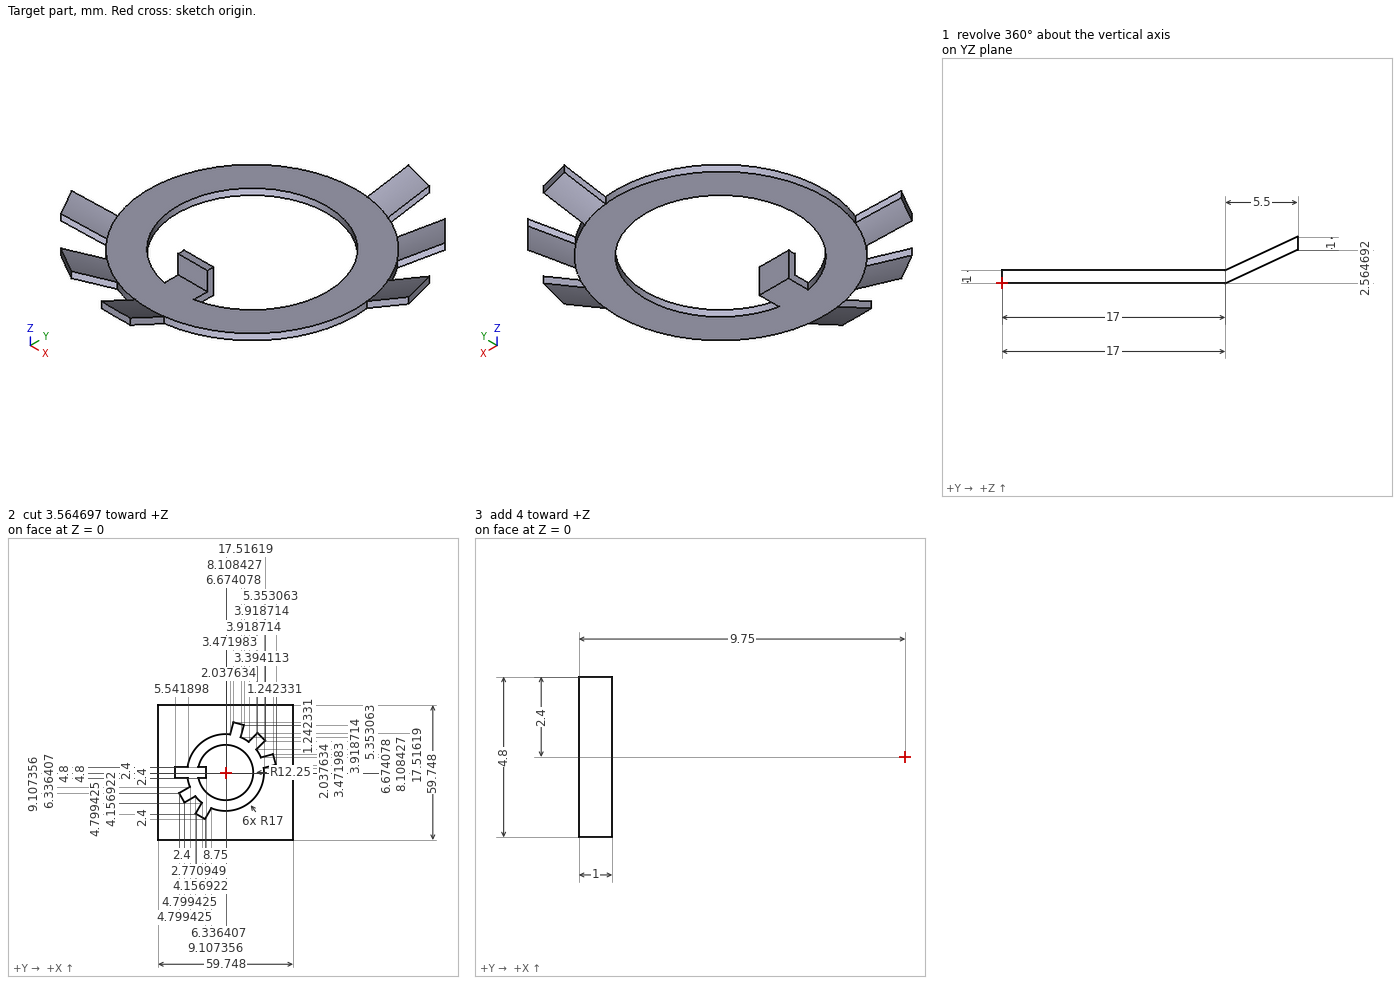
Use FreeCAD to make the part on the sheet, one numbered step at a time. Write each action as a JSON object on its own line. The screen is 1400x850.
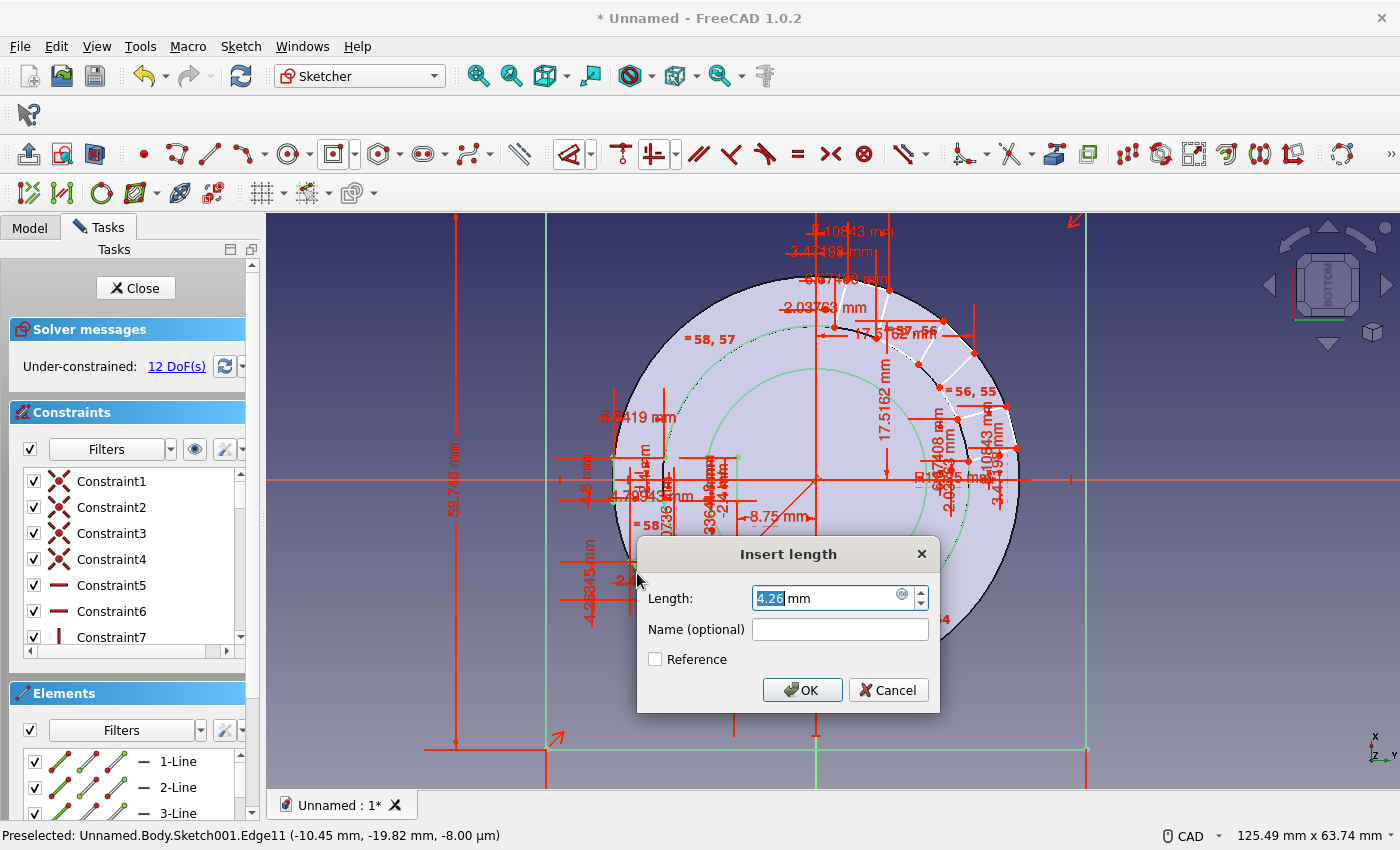
{"action": "type", "text": "4.156922"}
{"action": "key", "text": "Return"}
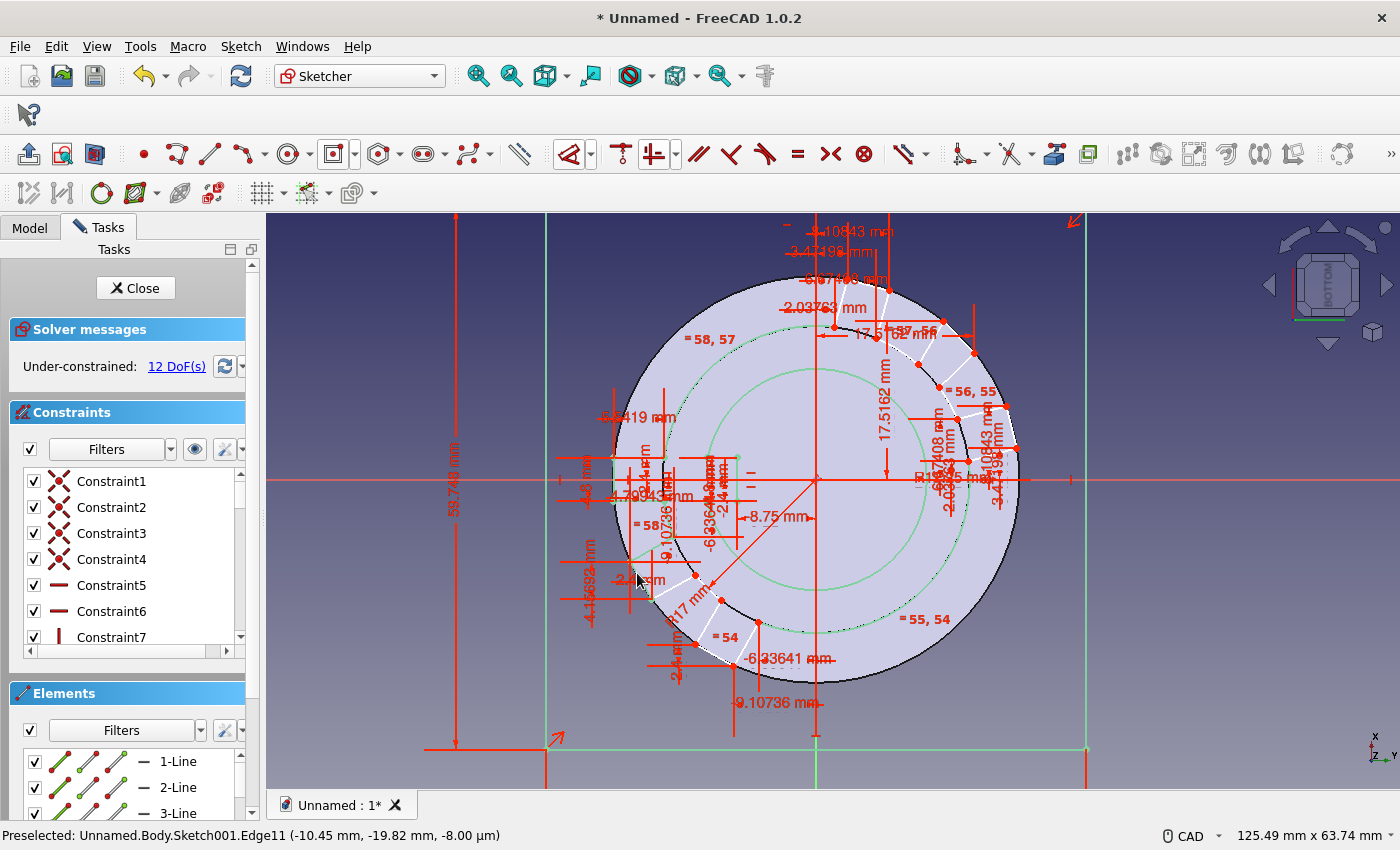
{"action": "left_click", "coordinate": [665, 592]}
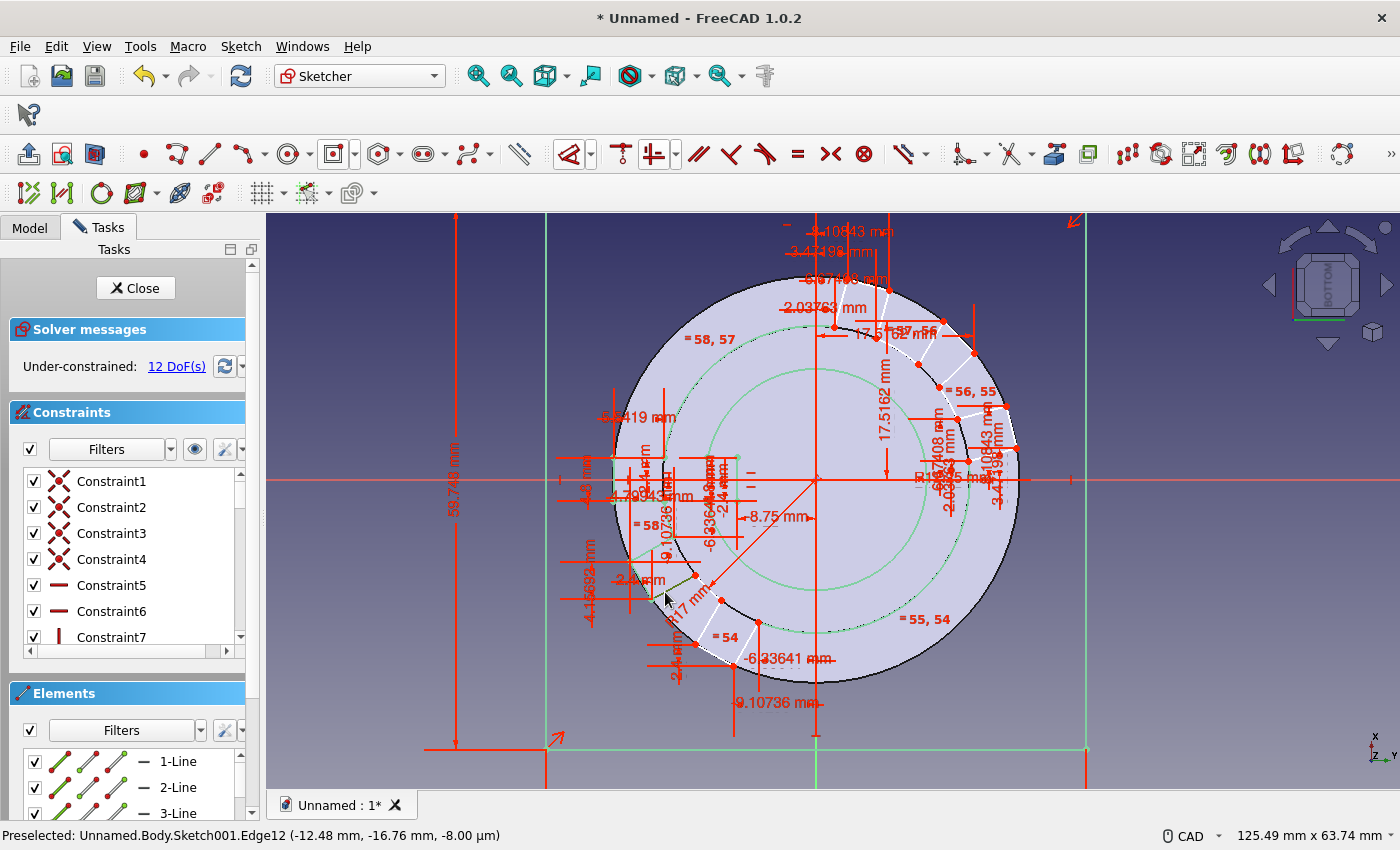
{"action": "left_click", "coordinate": [590, 154]}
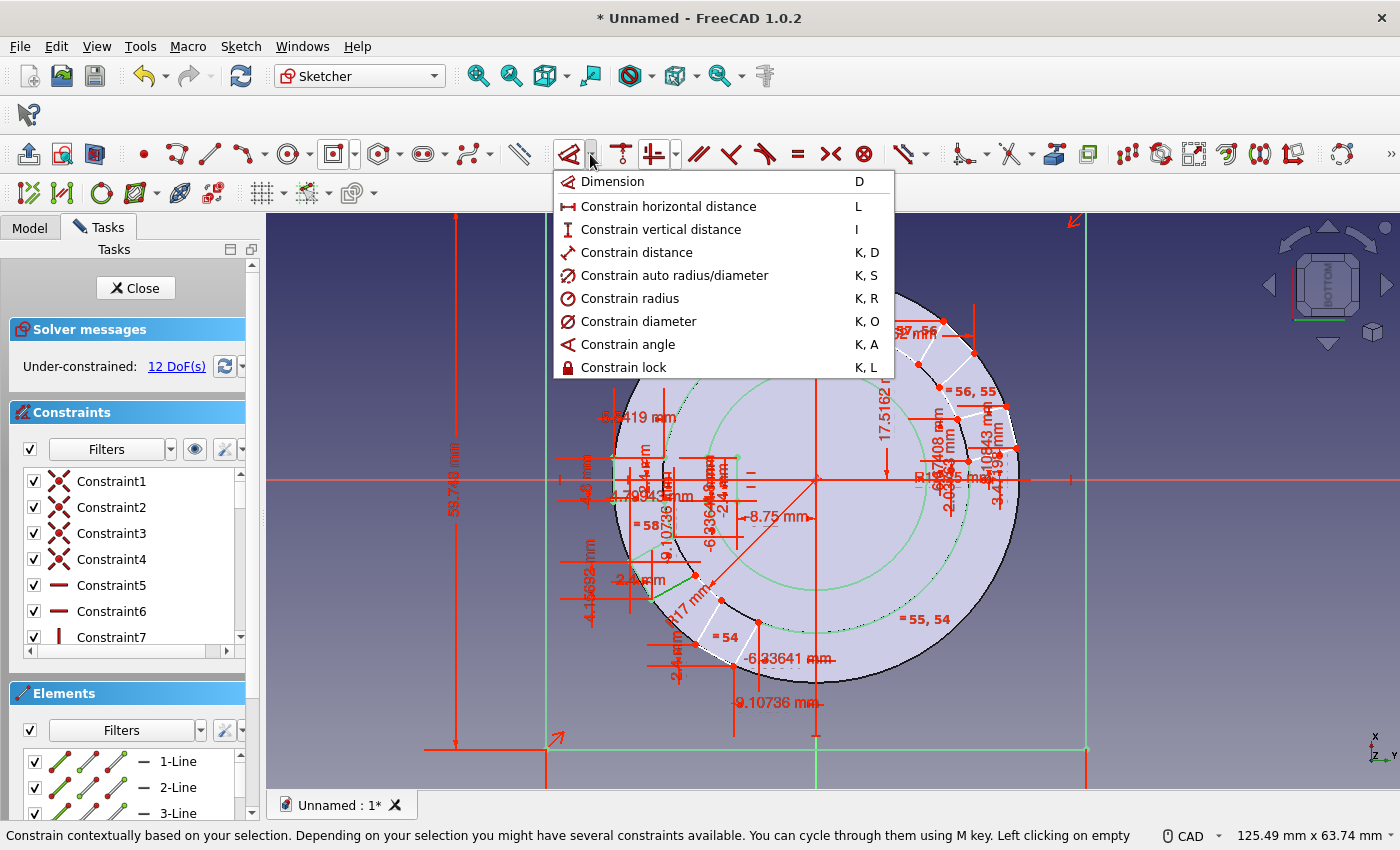
{"action": "left_click", "coordinate": [724, 206]}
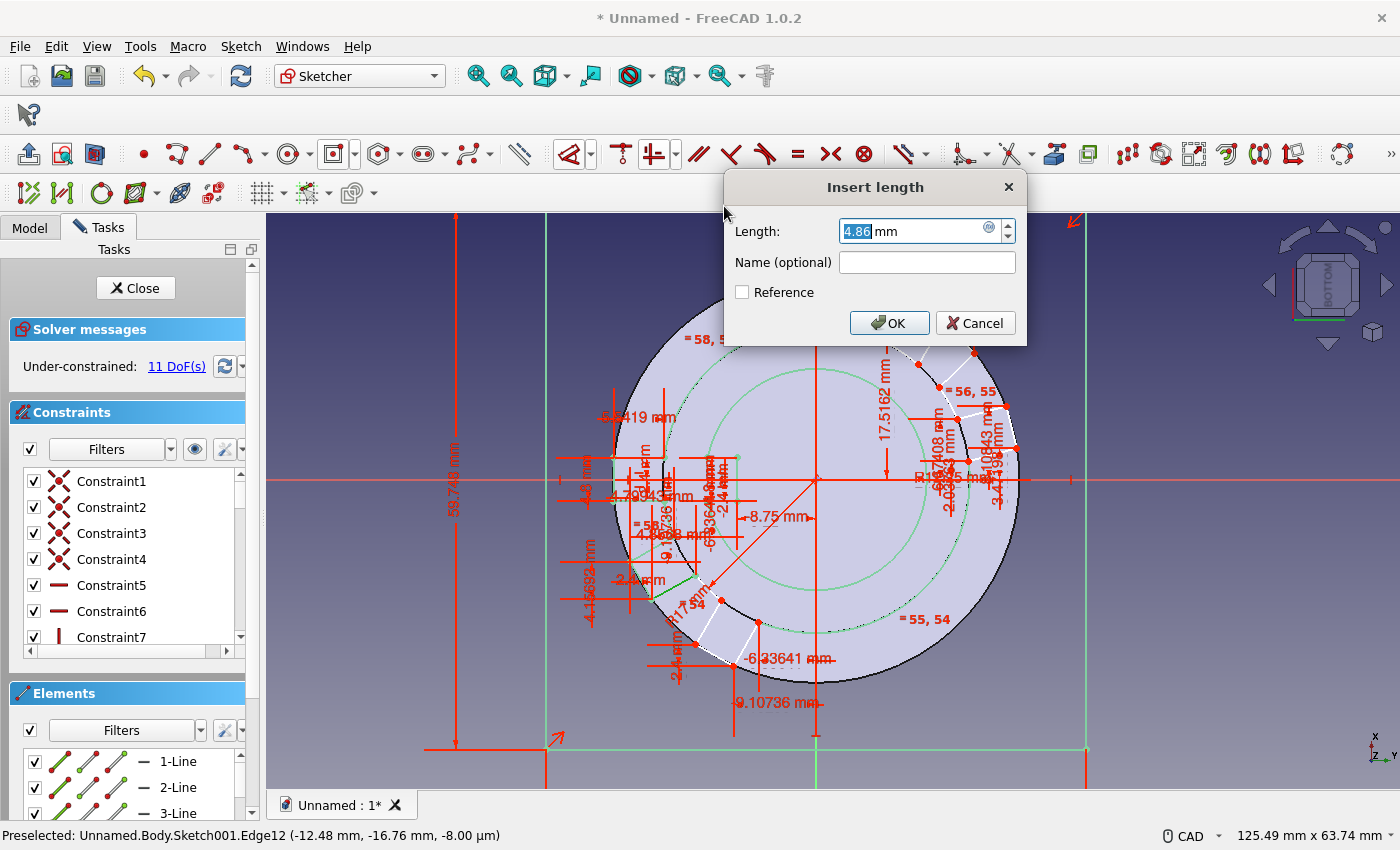
{"action": "type", "text": "4.799425"}
{"action": "key", "text": "Return"}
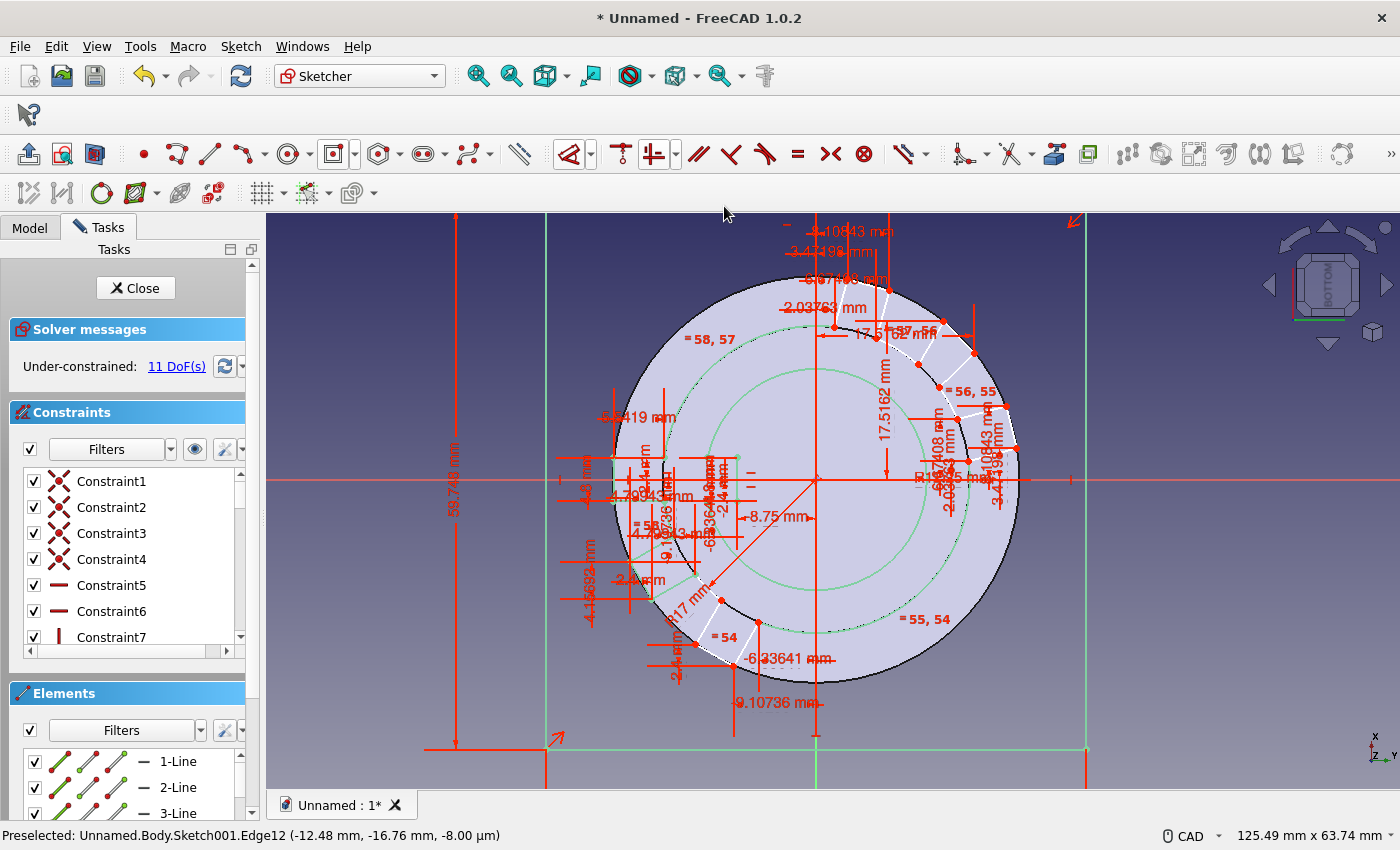
{"action": "scroll", "coordinate": [714, 614], "scroll_direction": "up", "scroll_amount": 3}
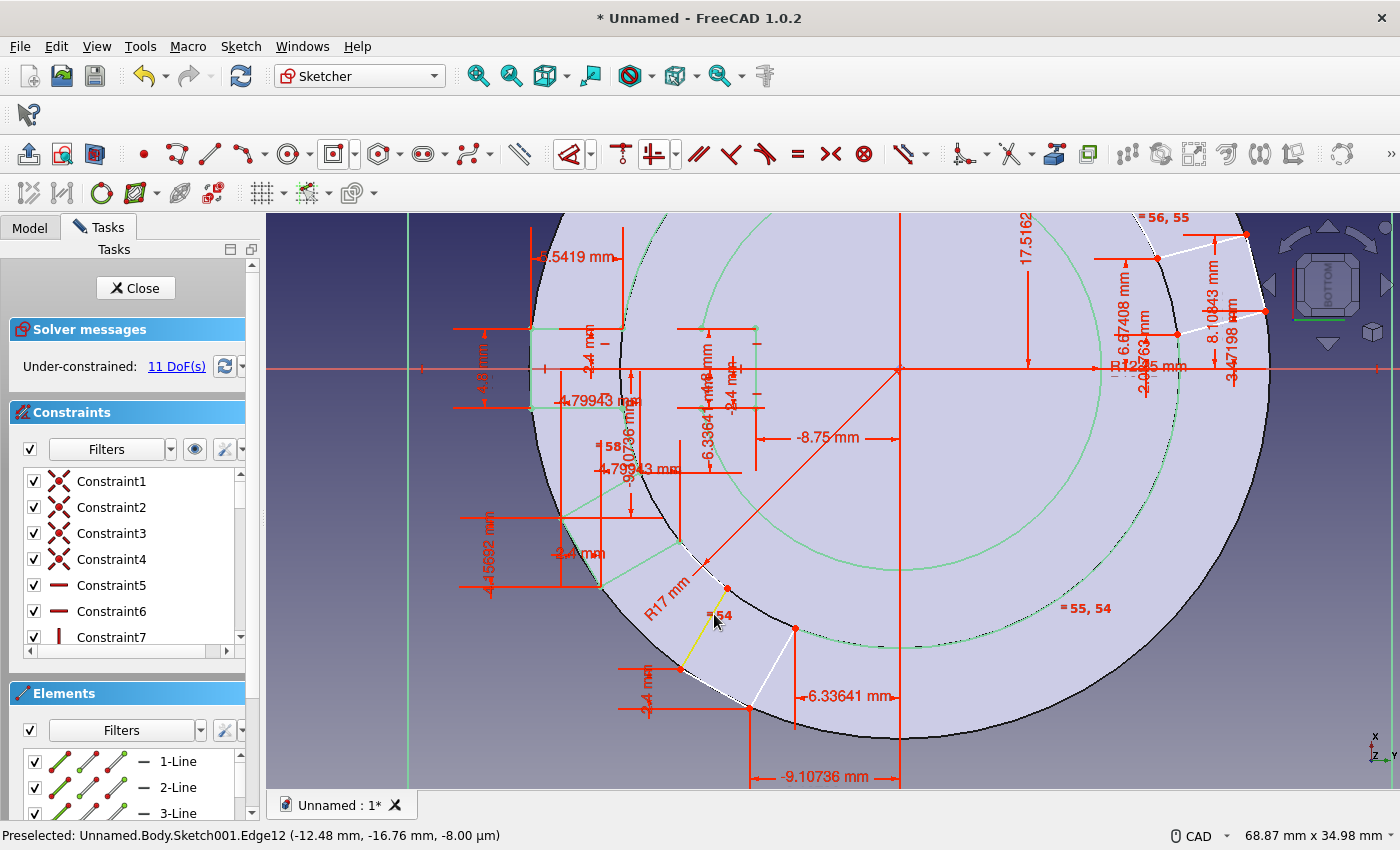
{"action": "left_click", "coordinate": [695, 645]}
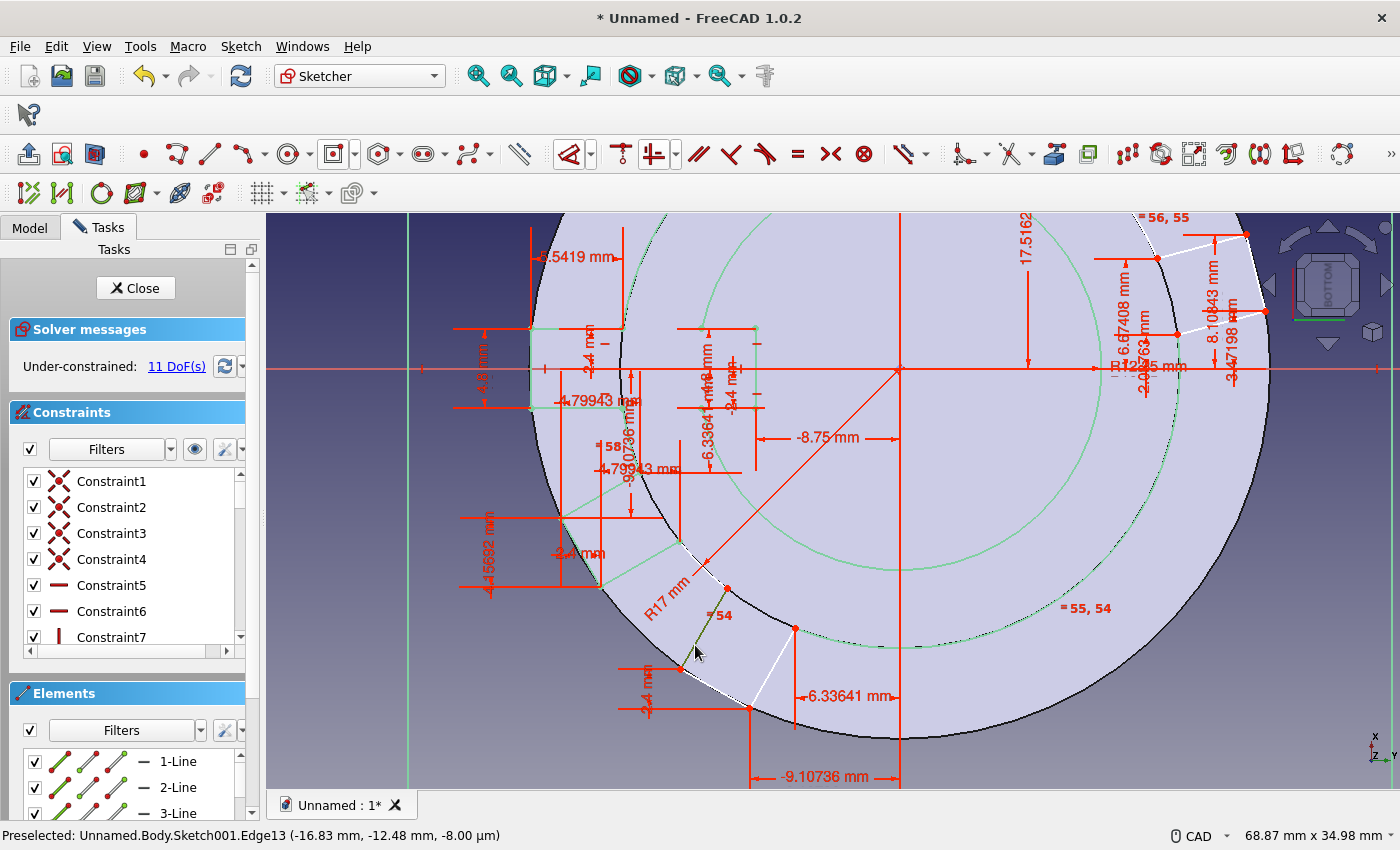
{"action": "key", "text": "l"}